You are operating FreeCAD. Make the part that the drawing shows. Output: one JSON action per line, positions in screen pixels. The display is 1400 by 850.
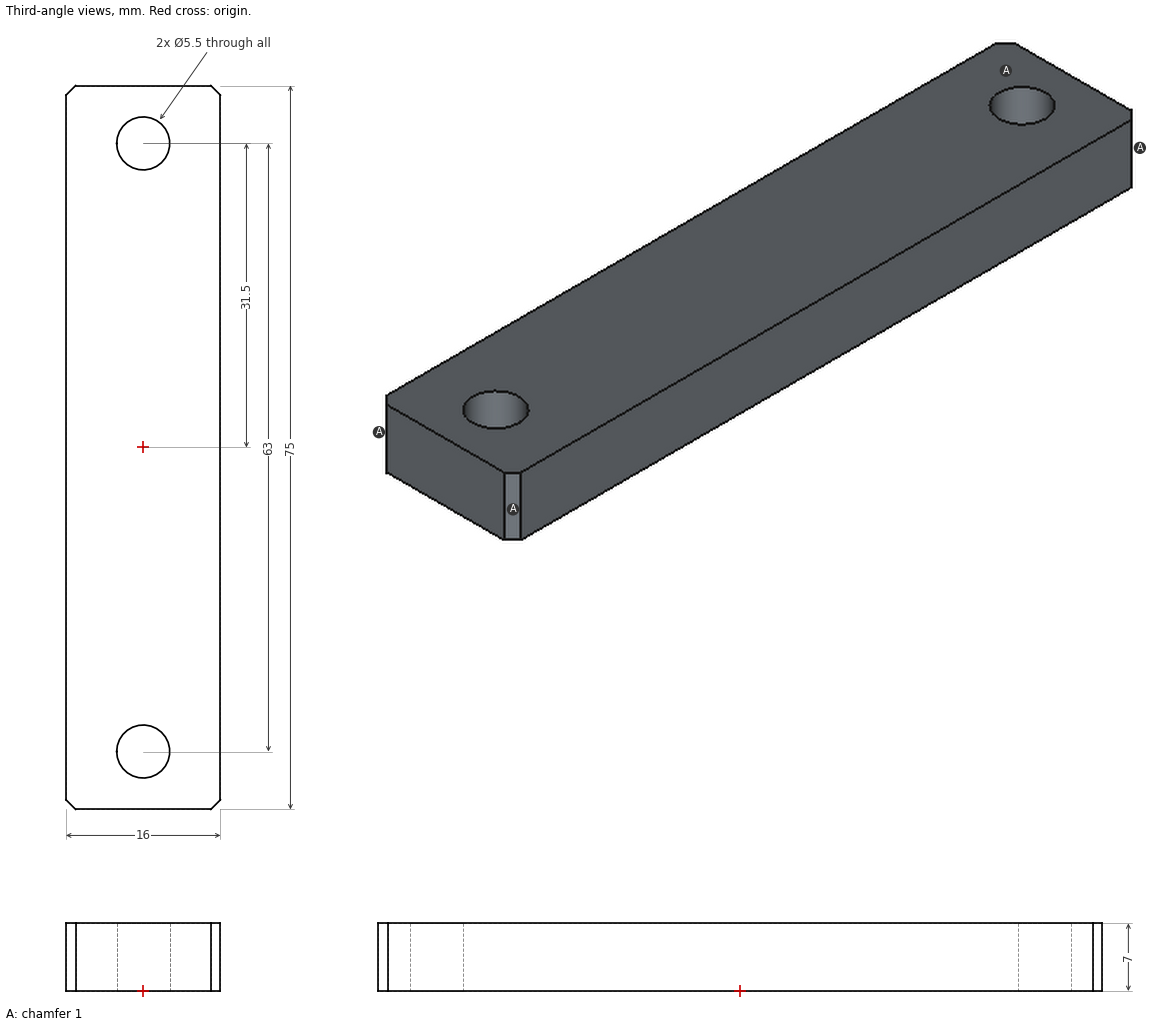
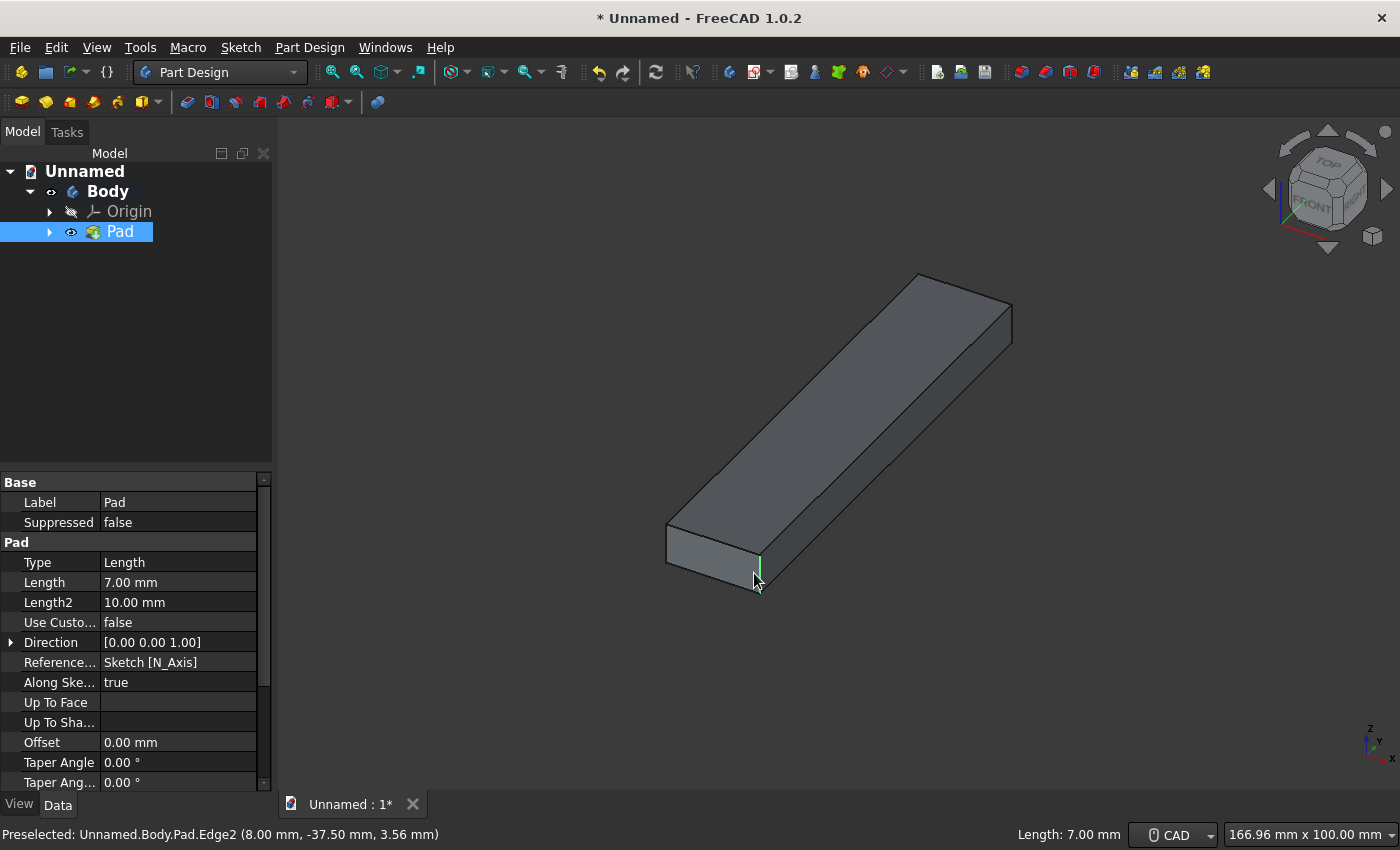
{"action": "key", "text": "0"}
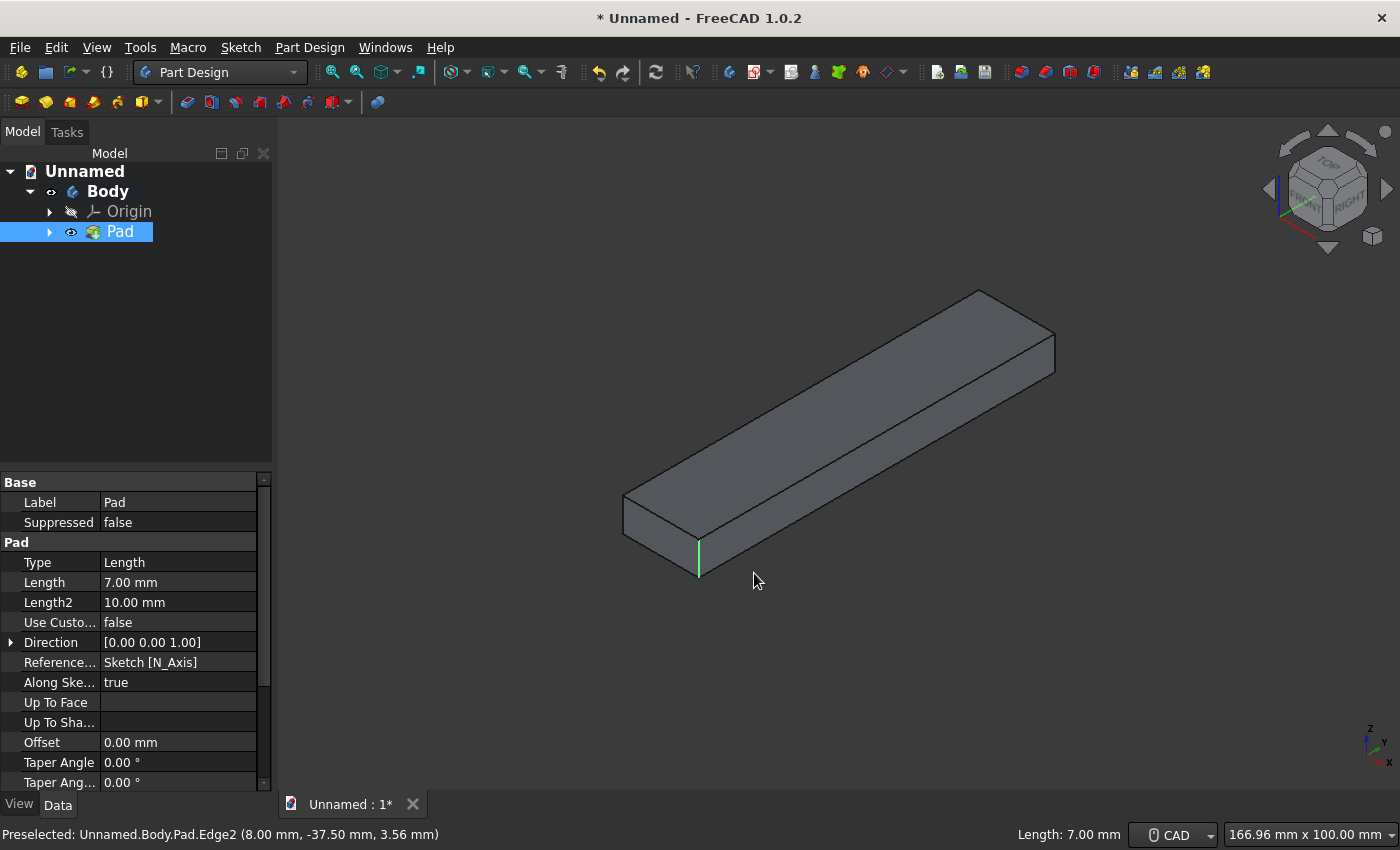
{"action": "left_click", "coordinate": [334, 72]}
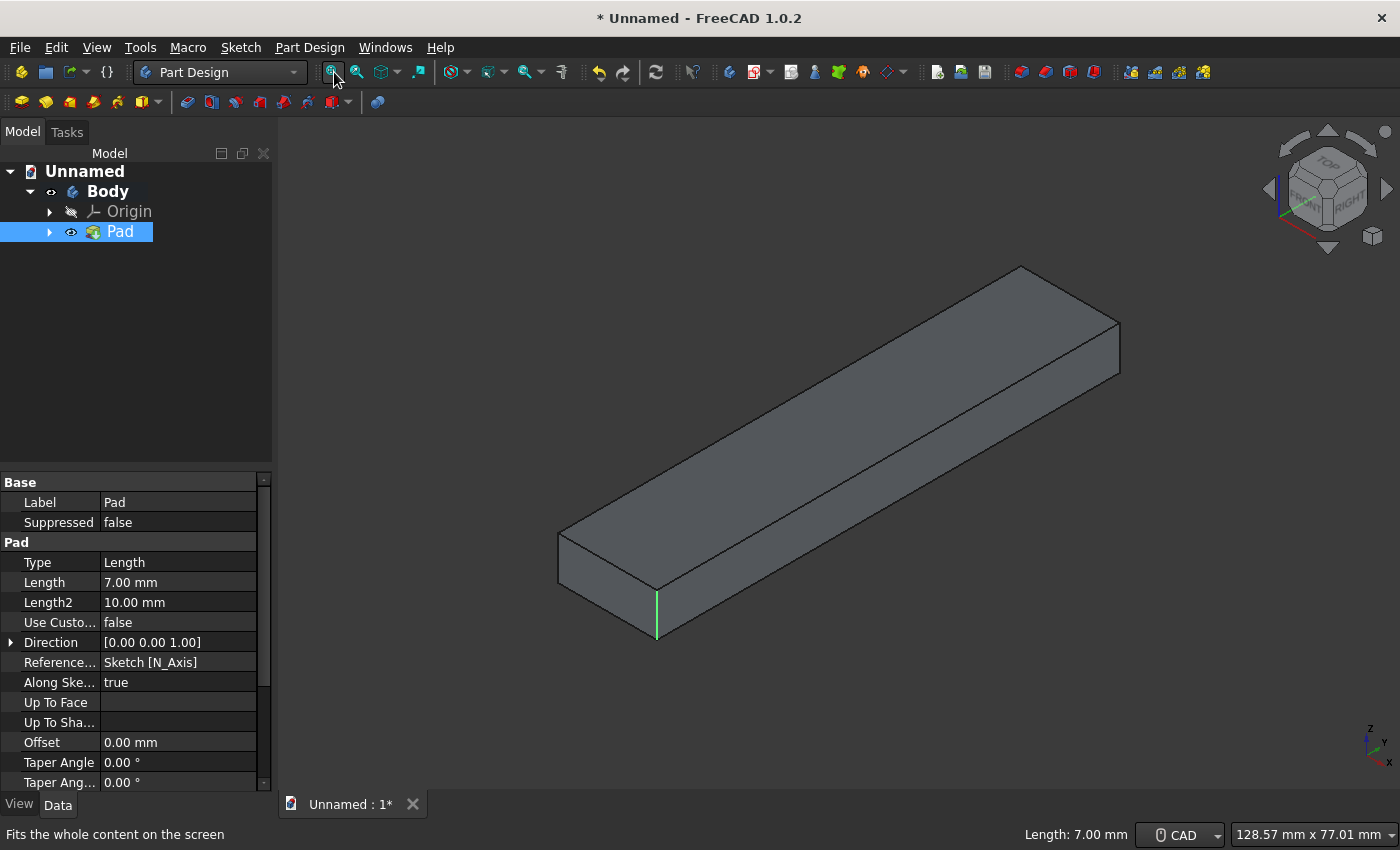
{"action": "key", "text": "2"}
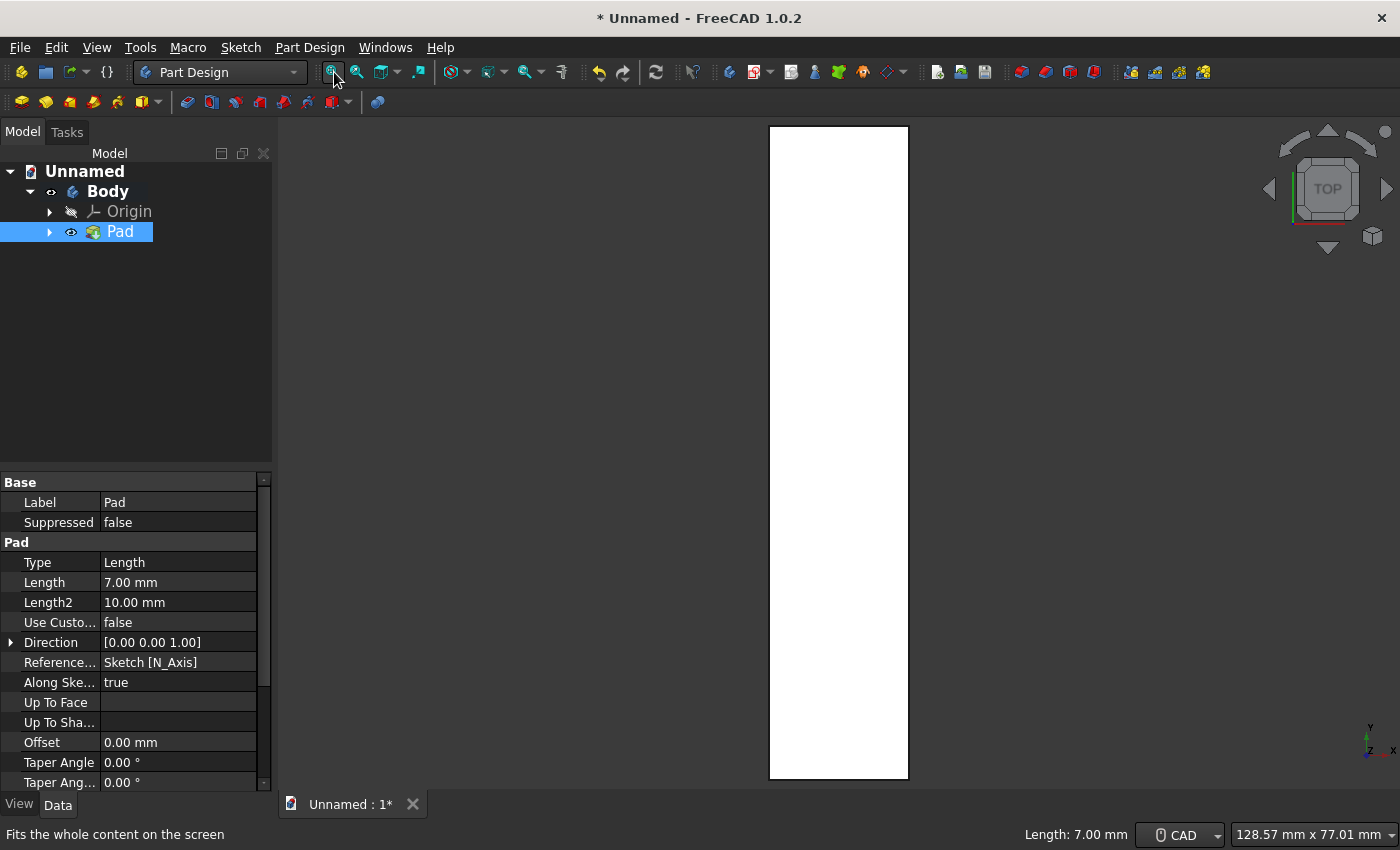
{"action": "key", "text": "1"}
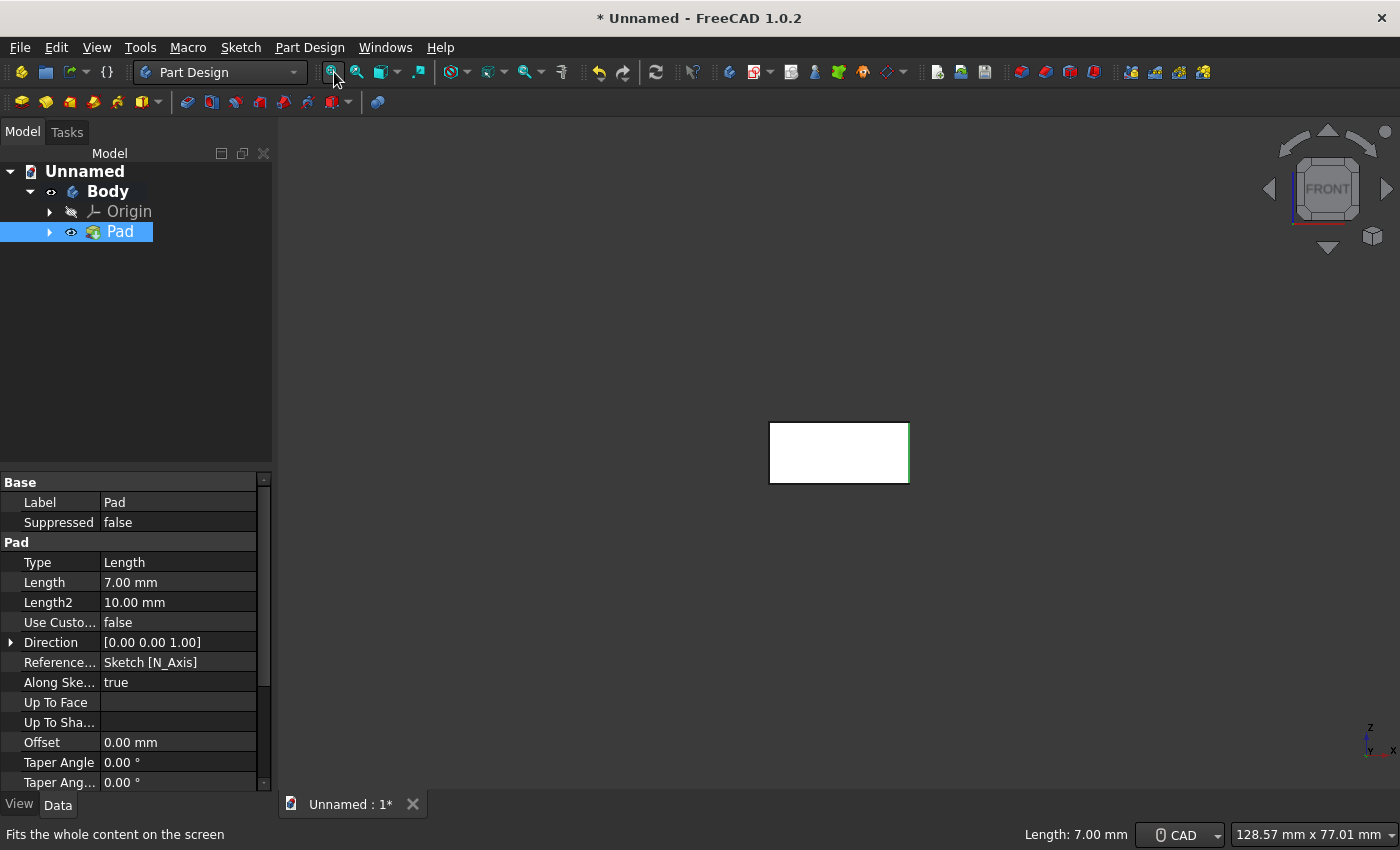
{"action": "key", "text": "v f"}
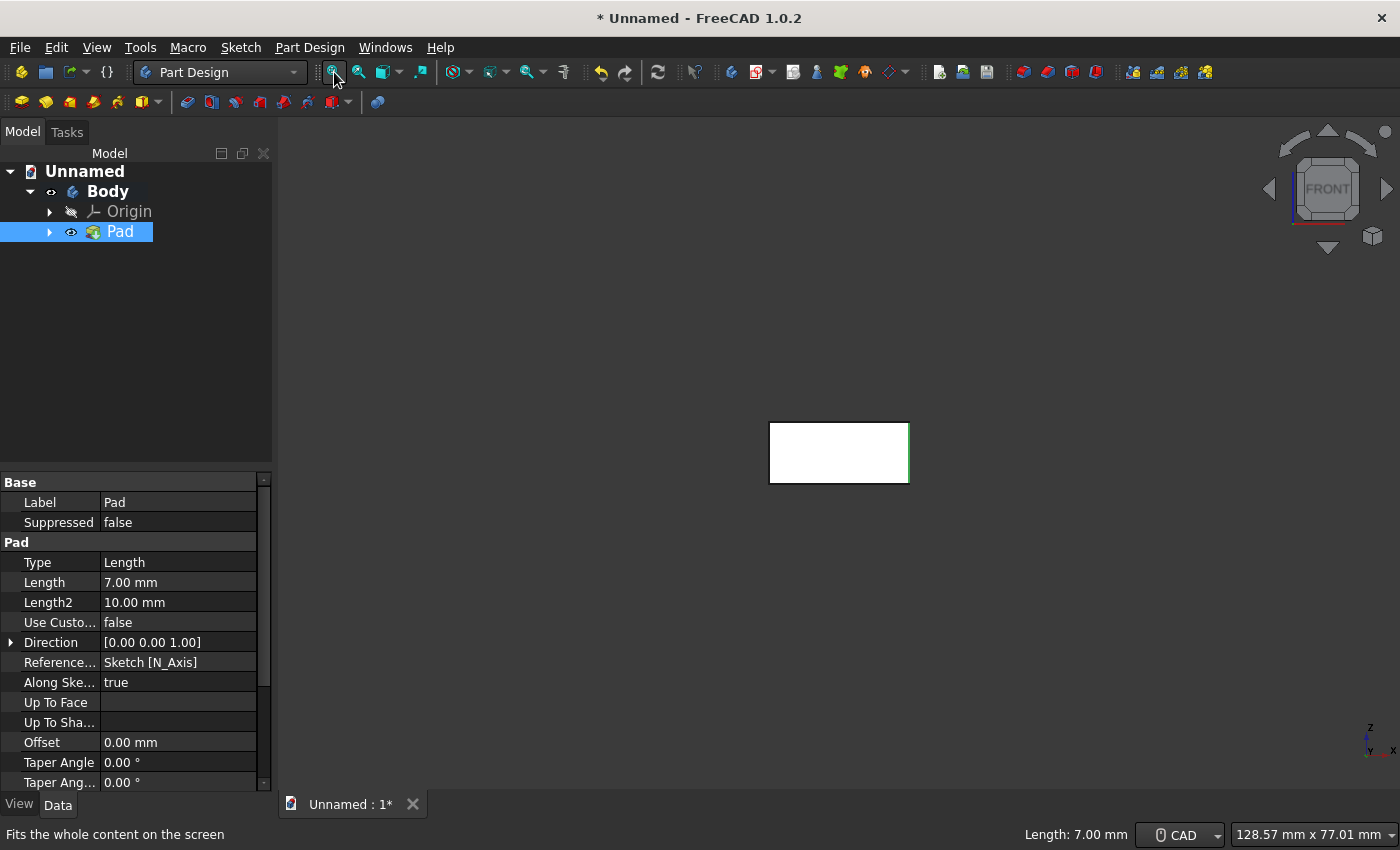
{"action": "left_click", "coordinate": [769, 452], "text": "ctrl"}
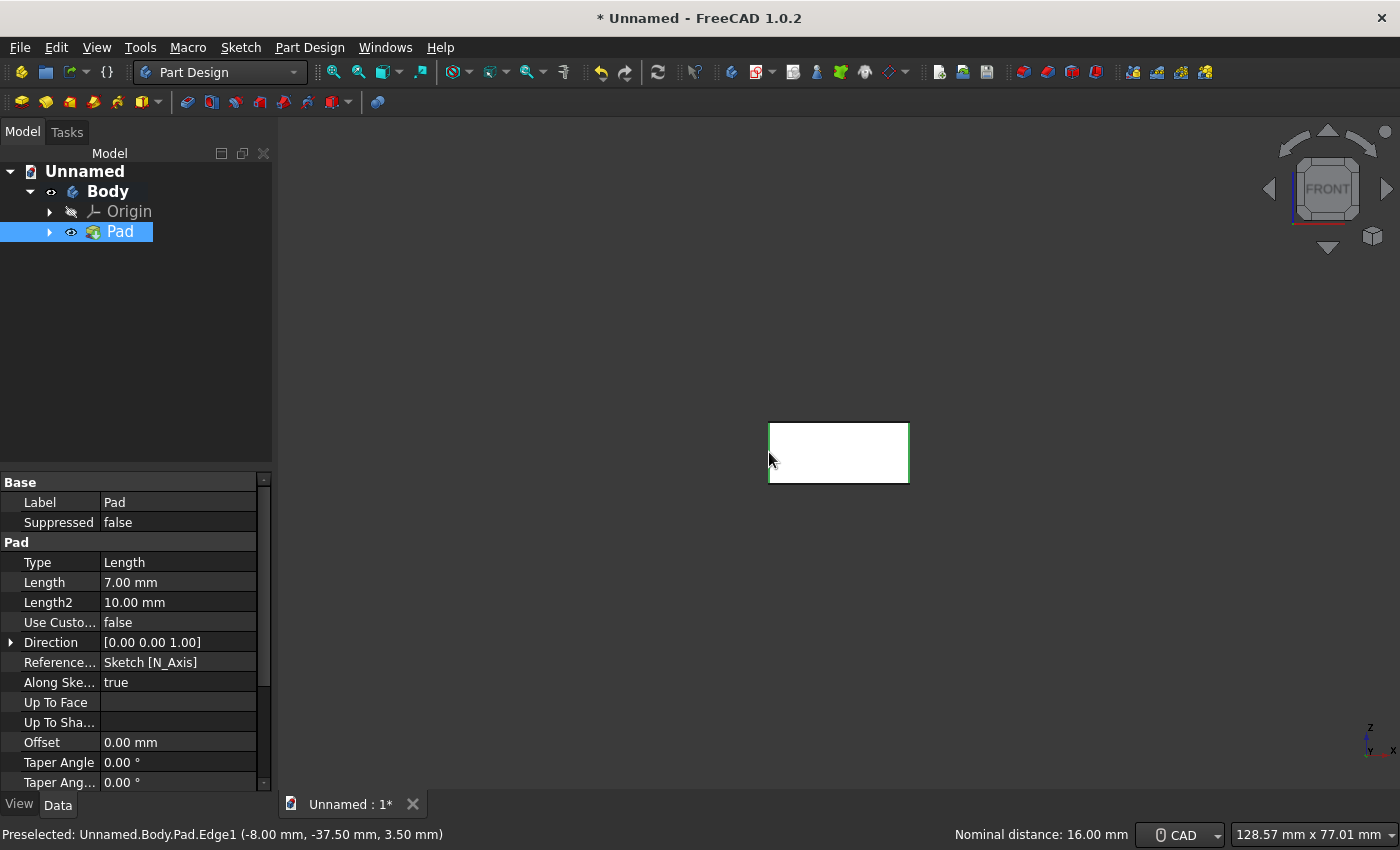
{"action": "key", "text": "3"}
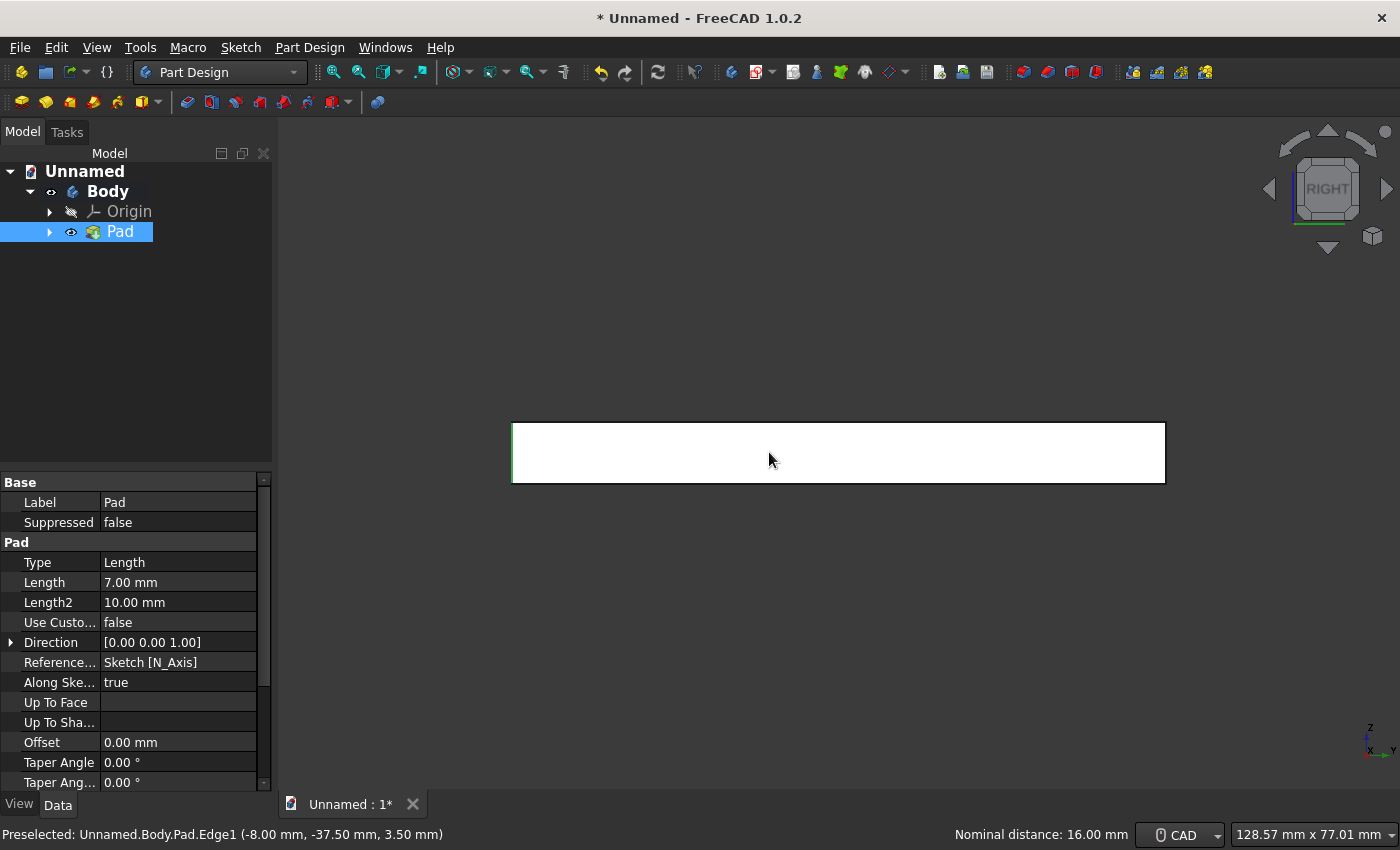
{"action": "left_click", "coordinate": [1166, 452], "text": "ctrl"}